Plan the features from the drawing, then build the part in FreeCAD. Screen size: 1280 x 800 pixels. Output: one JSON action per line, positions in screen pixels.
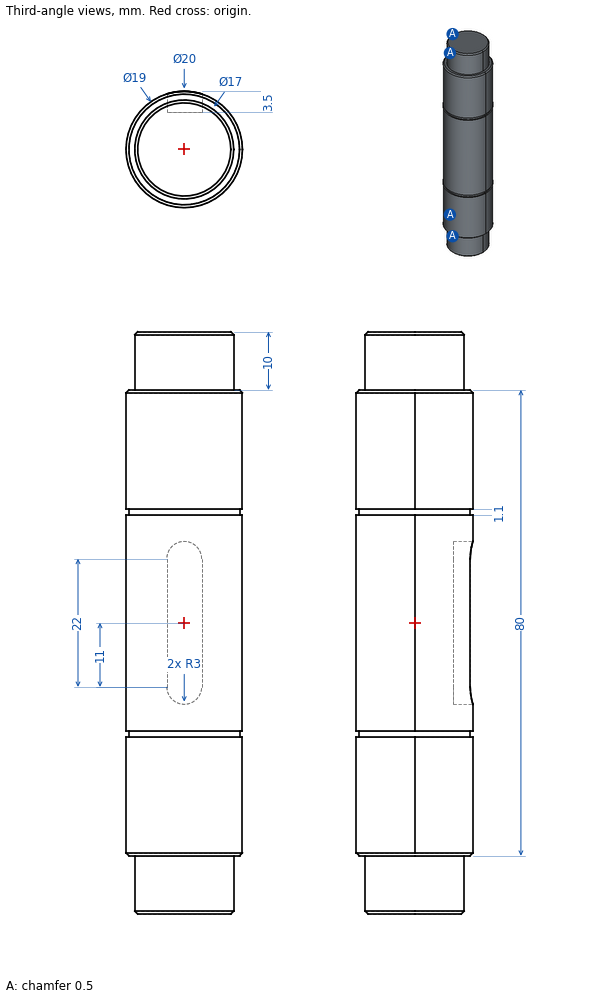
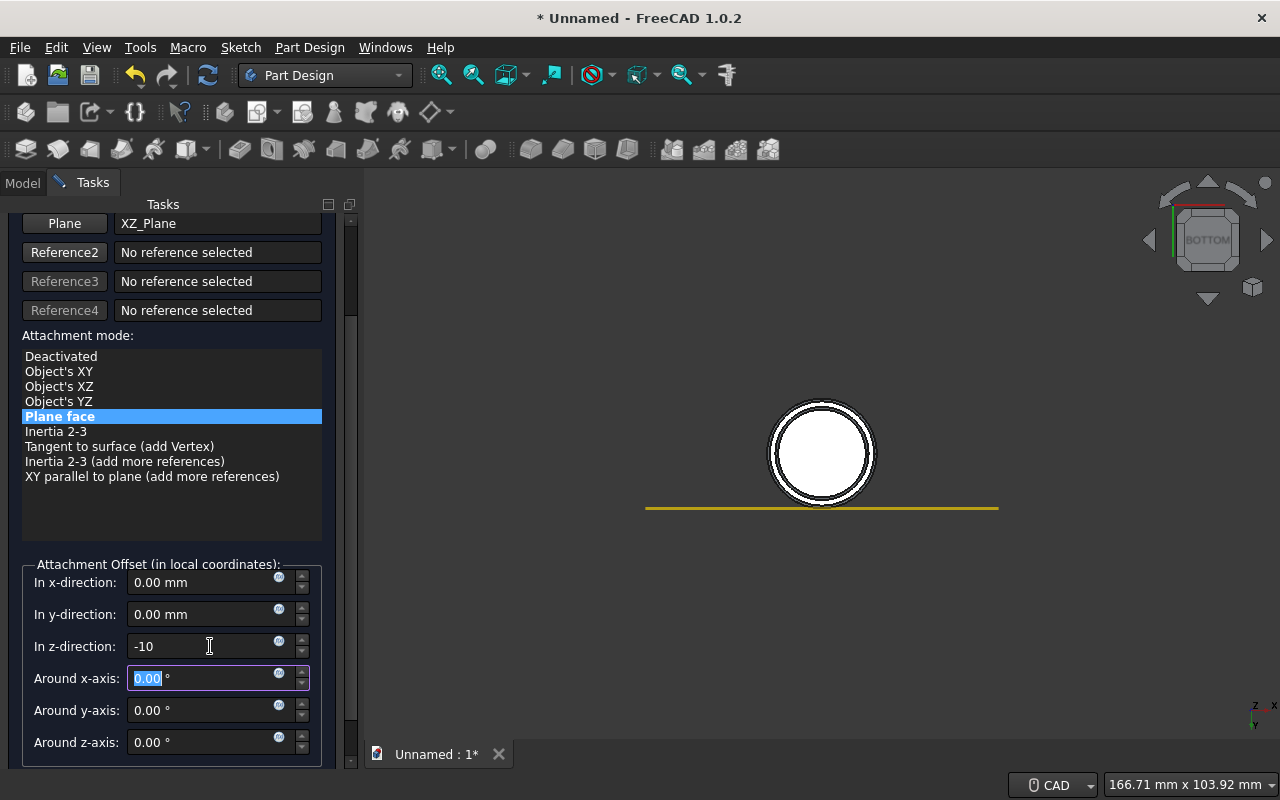
{"action": "scroll", "coordinate": [351, 491], "scroll_direction": "up", "scroll_amount": 3}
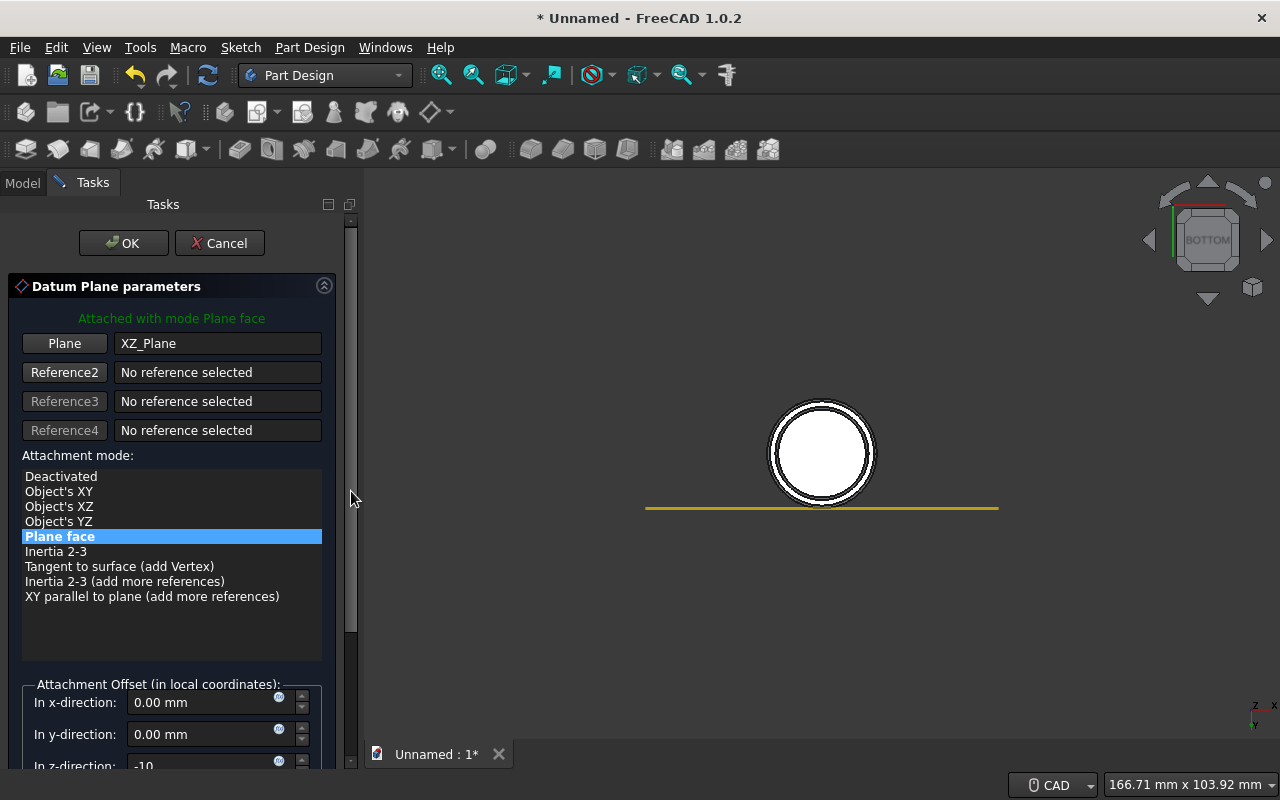
{"action": "left_click", "coordinate": [124, 243]}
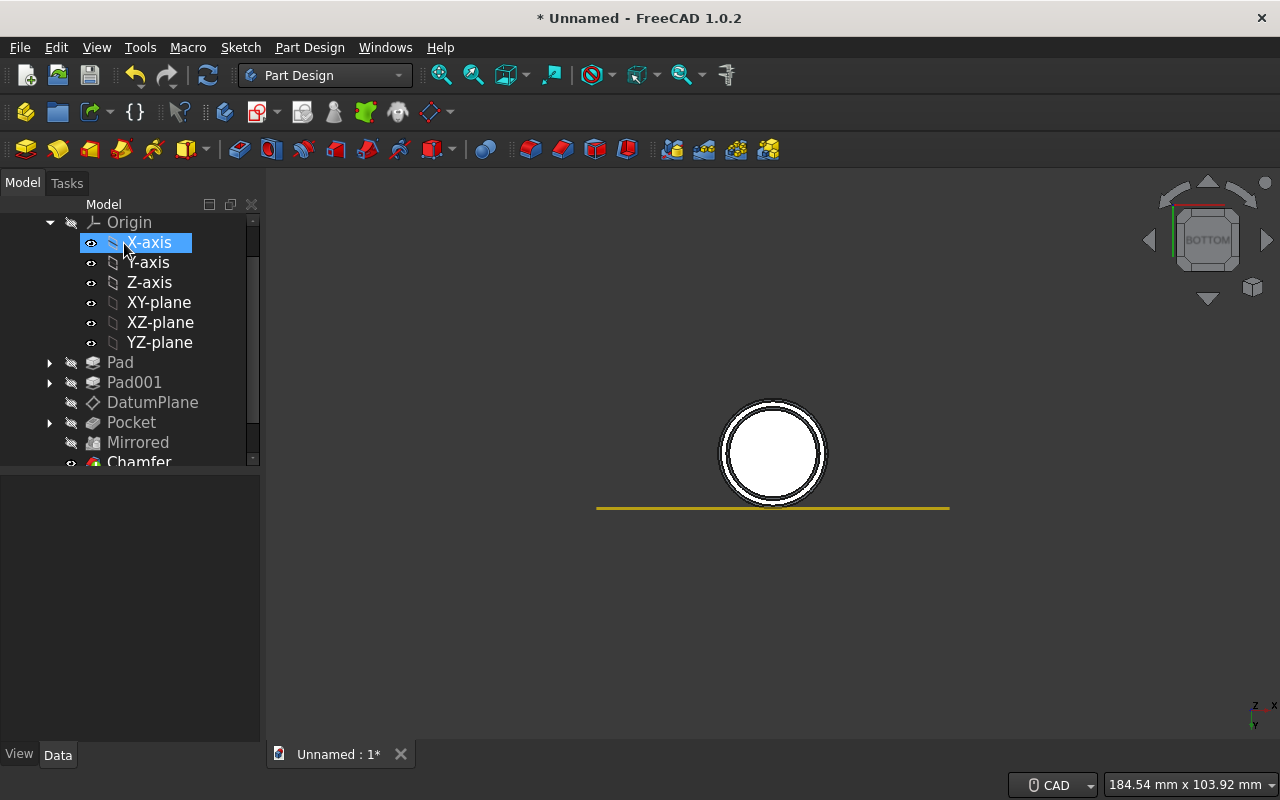
{"action": "scroll", "coordinate": [140, 338], "scroll_direction": "down", "scroll_amount": 3}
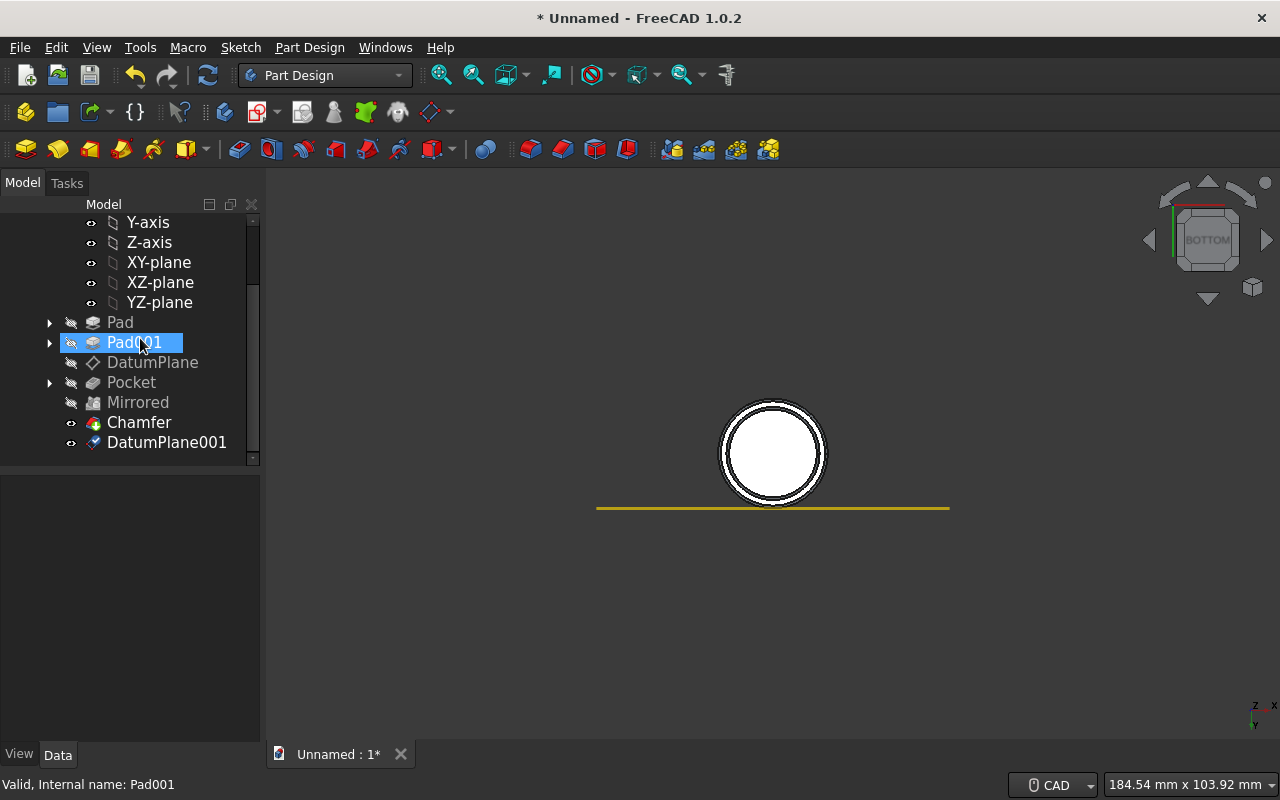
{"action": "left_click", "coordinate": [116, 443]}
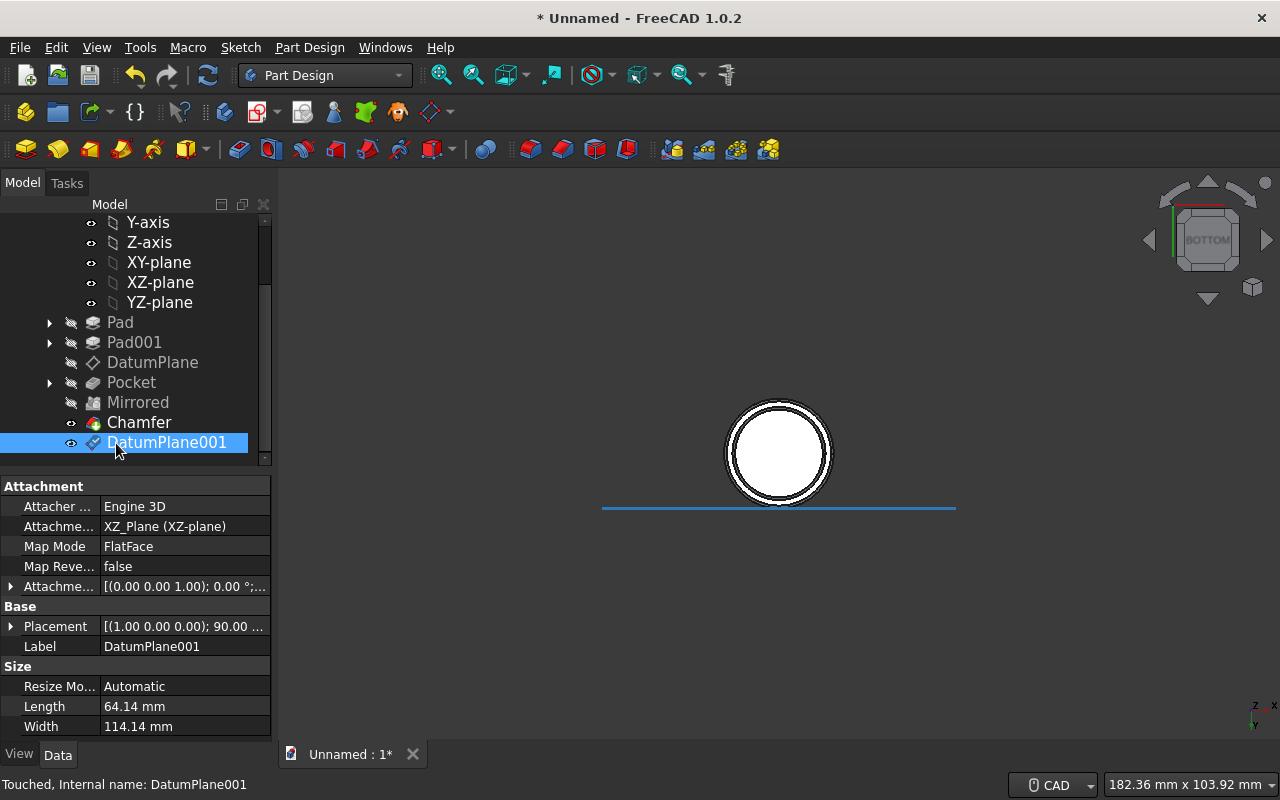
{"action": "left_click", "coordinate": [258, 112]}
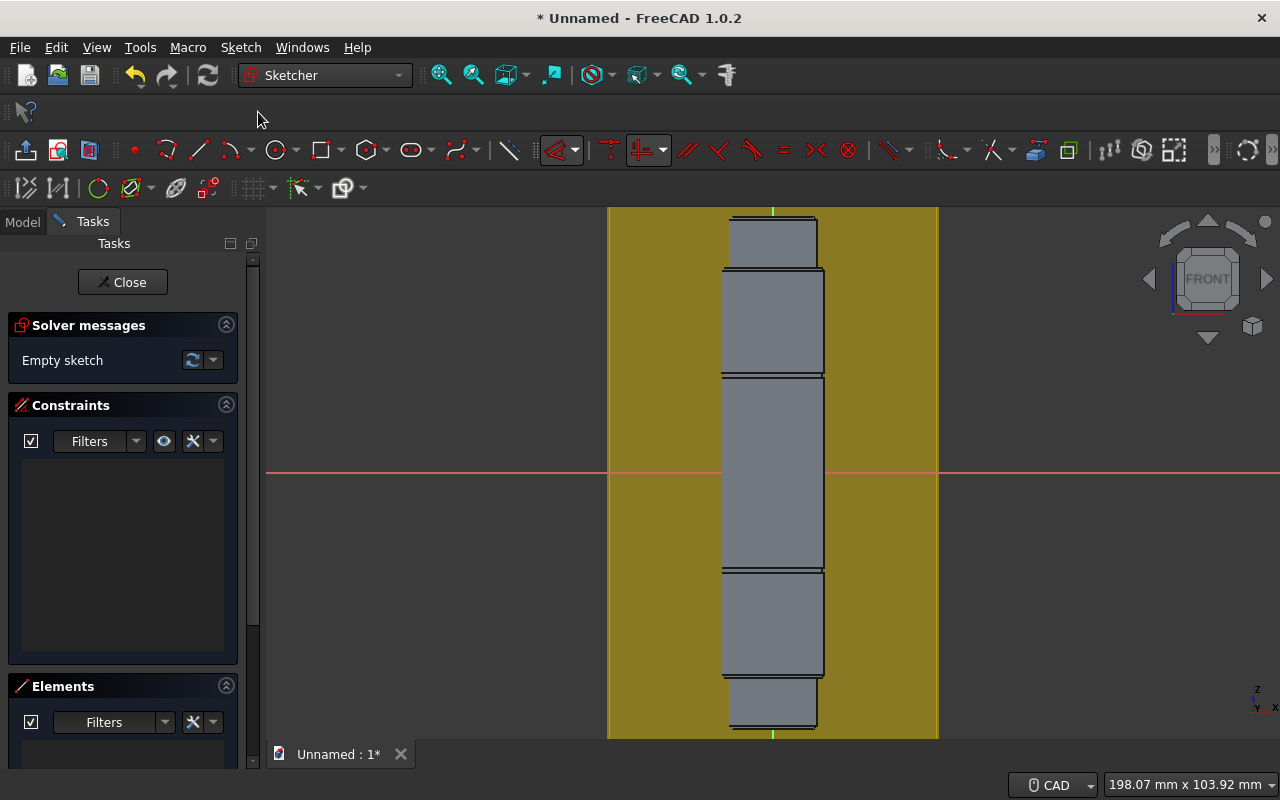
{"action": "key", "text": "q s"}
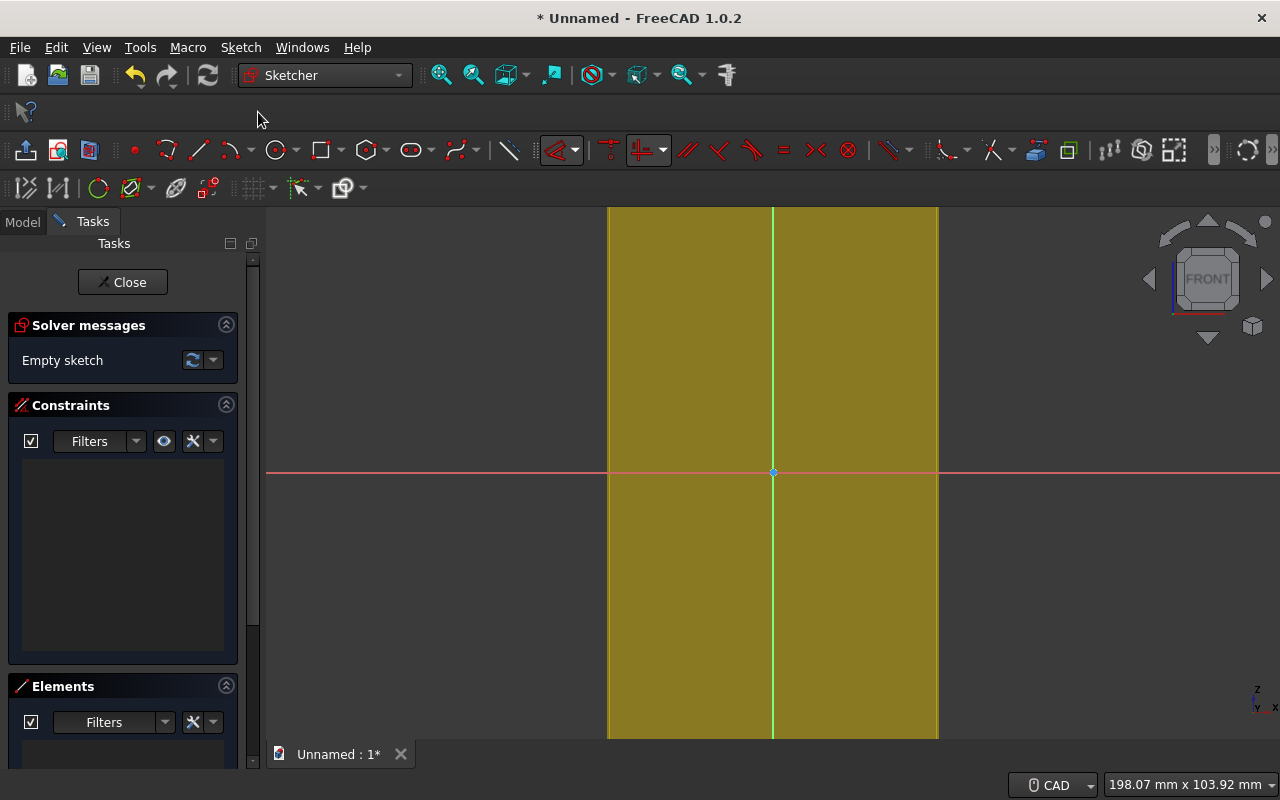
{"action": "scroll", "coordinate": [829, 473], "scroll_direction": "up", "scroll_amount": 4}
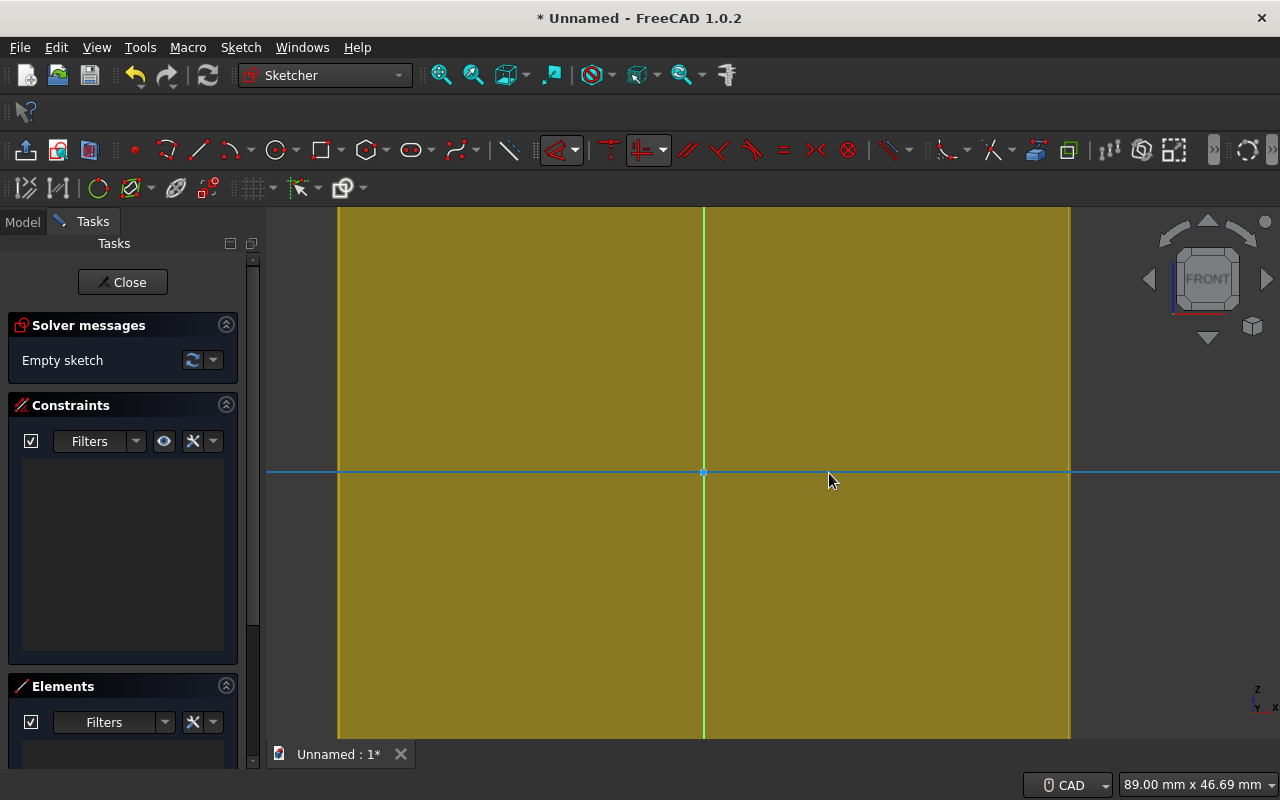
{"action": "key", "text": "g s"}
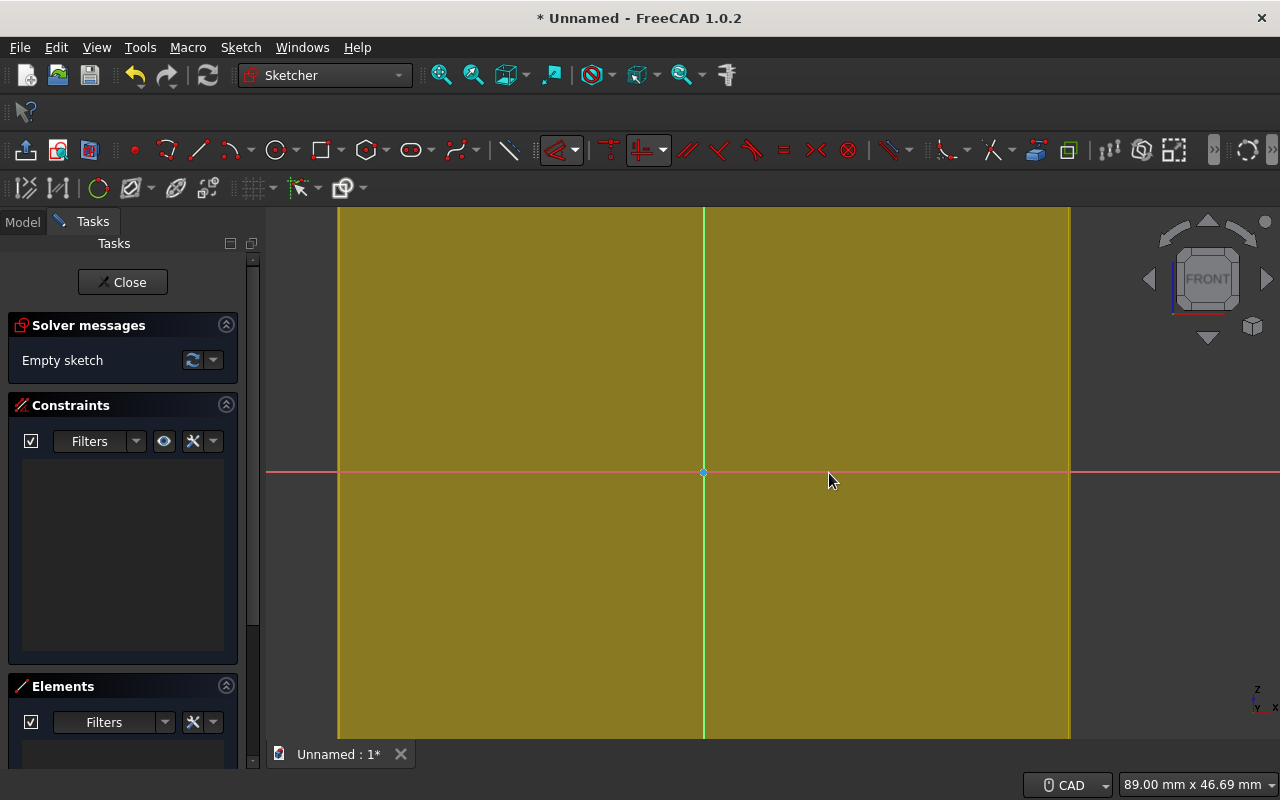
{"action": "left_click", "coordinate": [704, 598]}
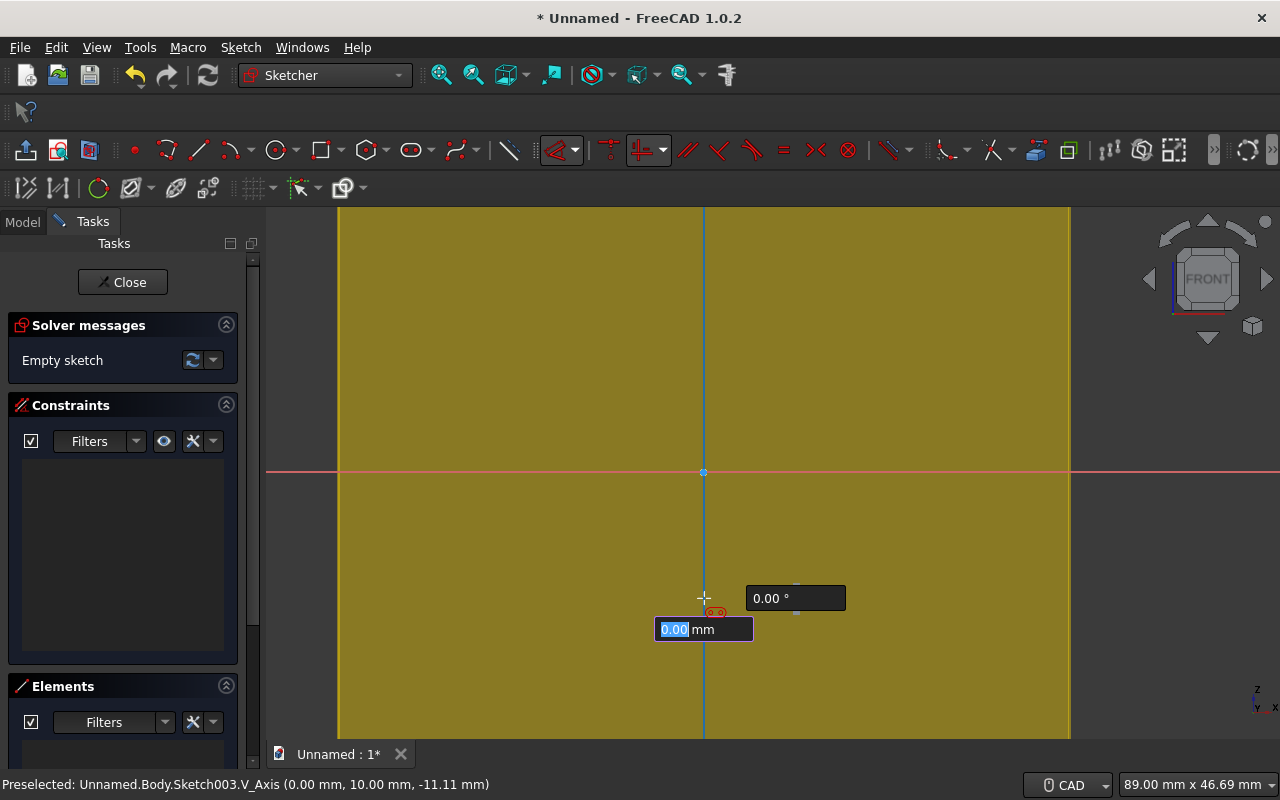
{"action": "left_click", "coordinate": [713, 347]}